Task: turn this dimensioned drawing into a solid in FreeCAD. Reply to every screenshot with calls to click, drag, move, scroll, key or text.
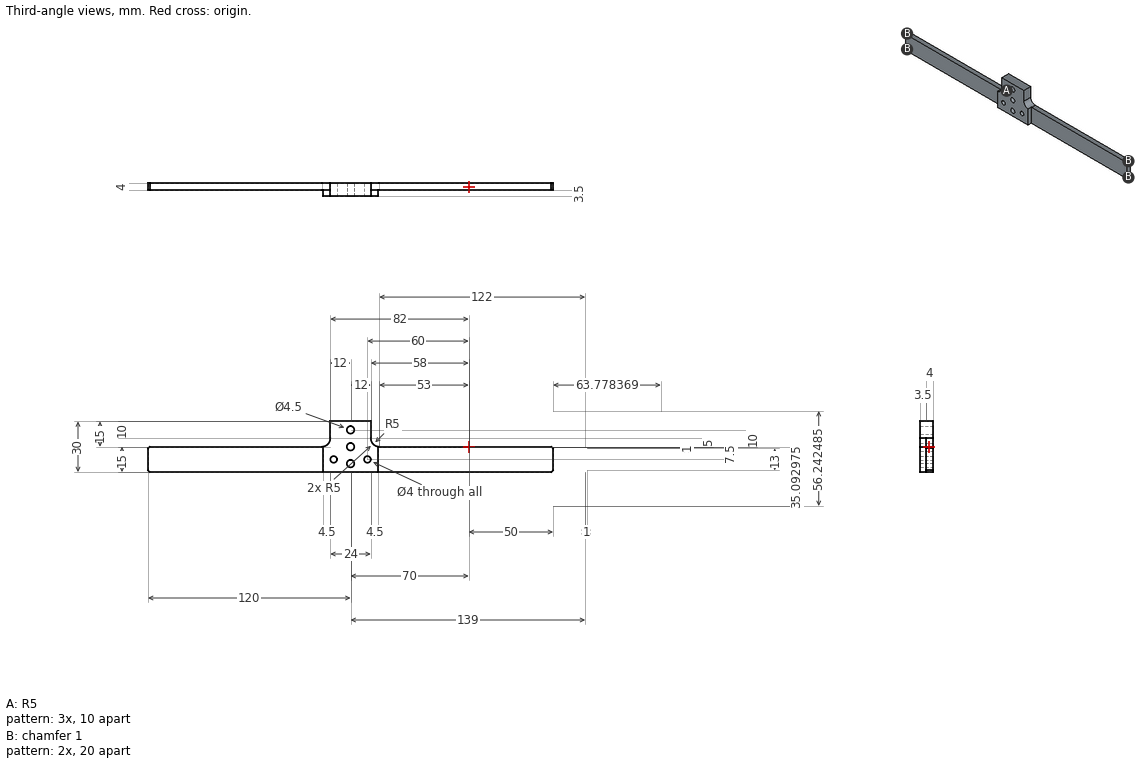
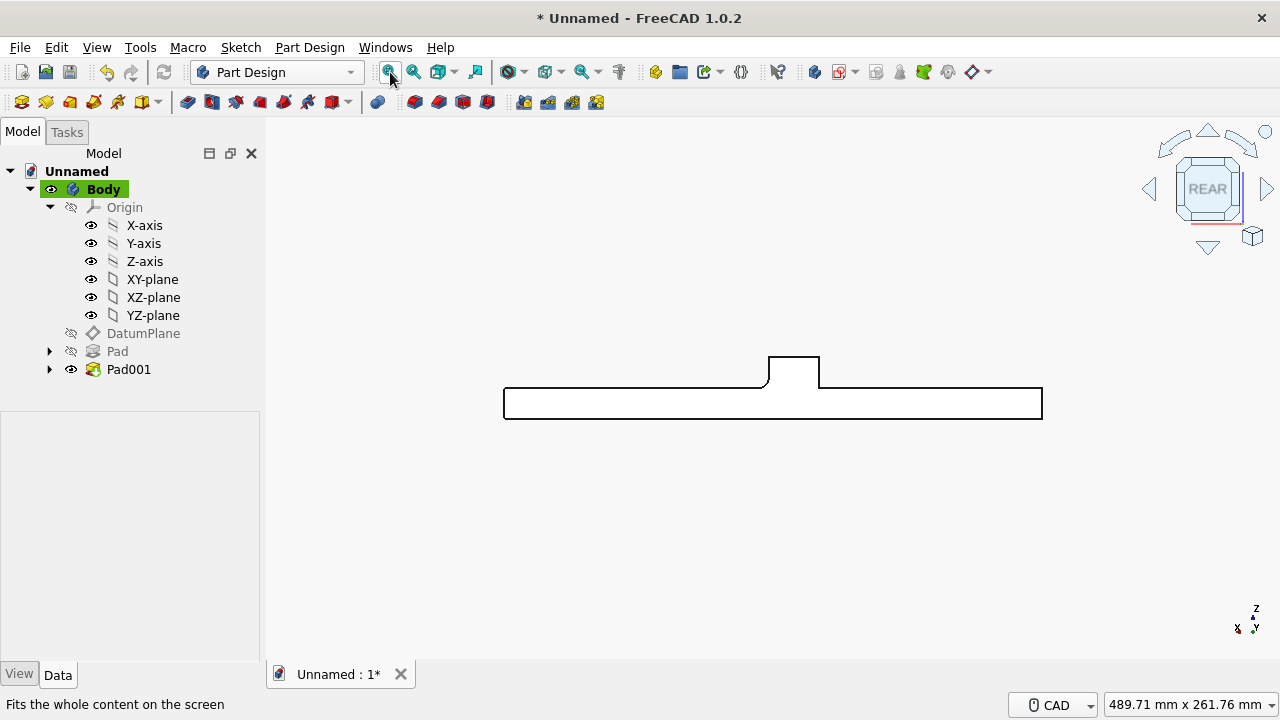
scroll(819, 387, up, 8)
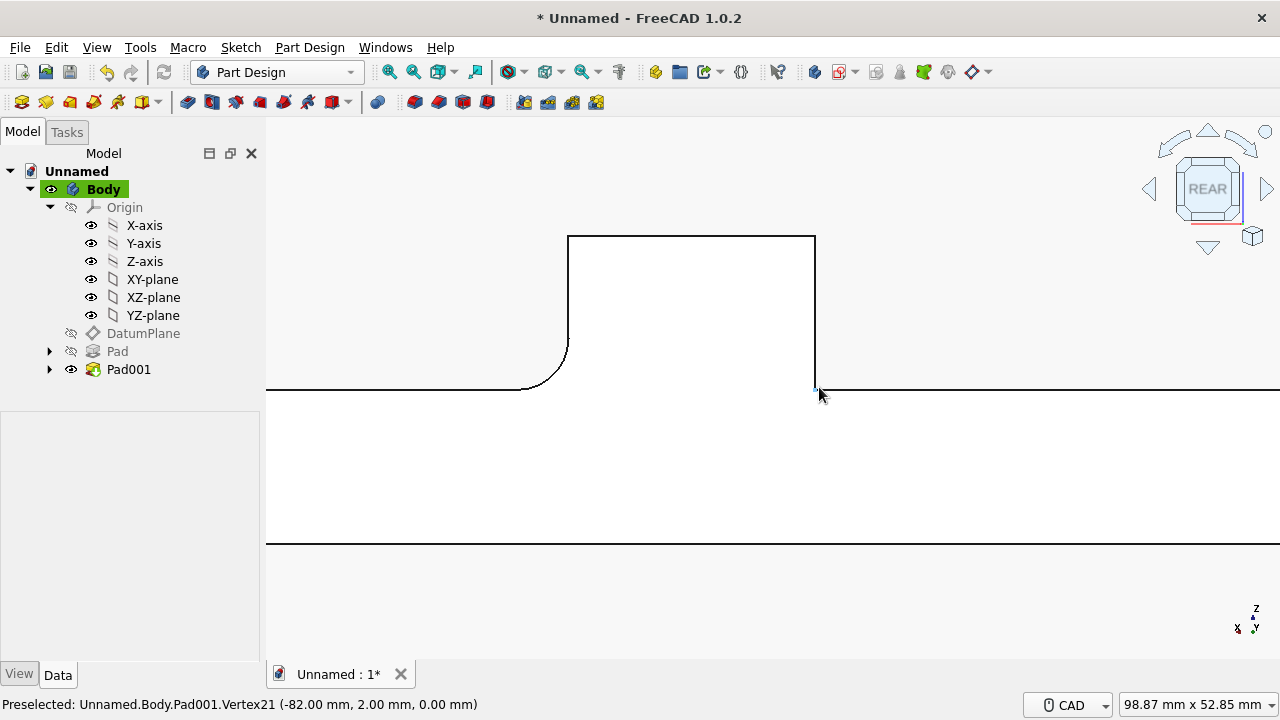
click(390, 72)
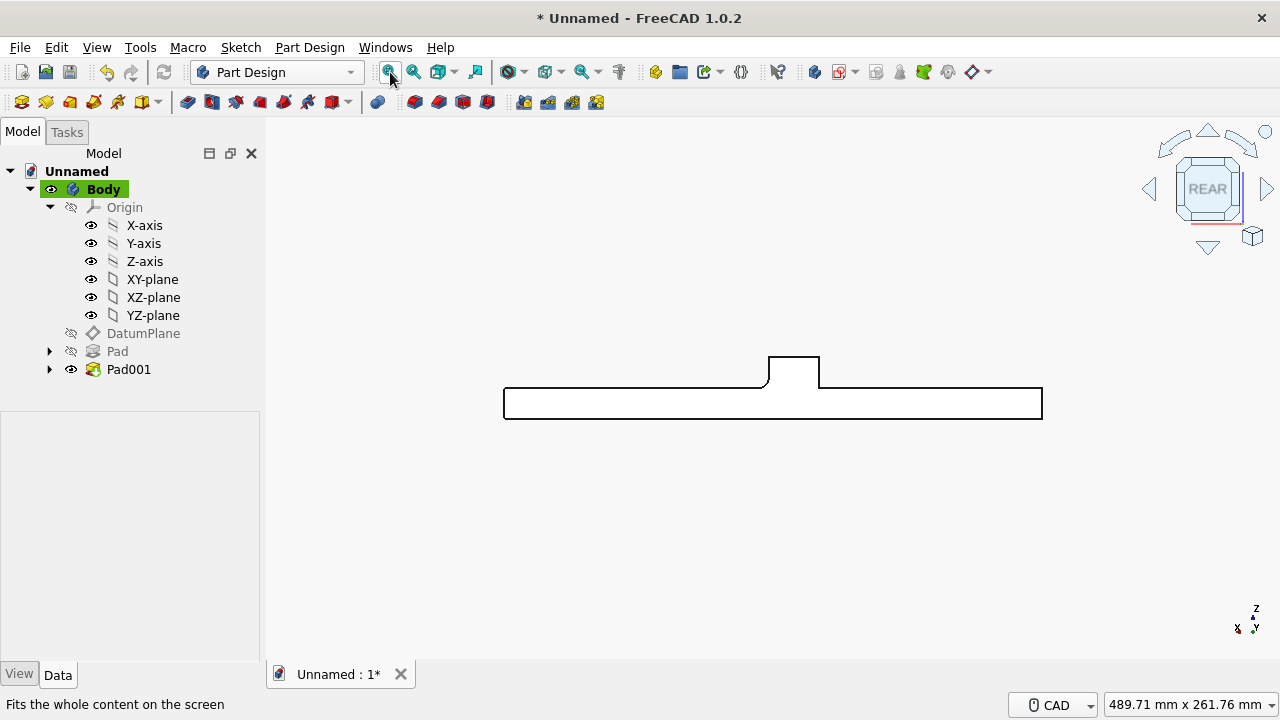
key(6)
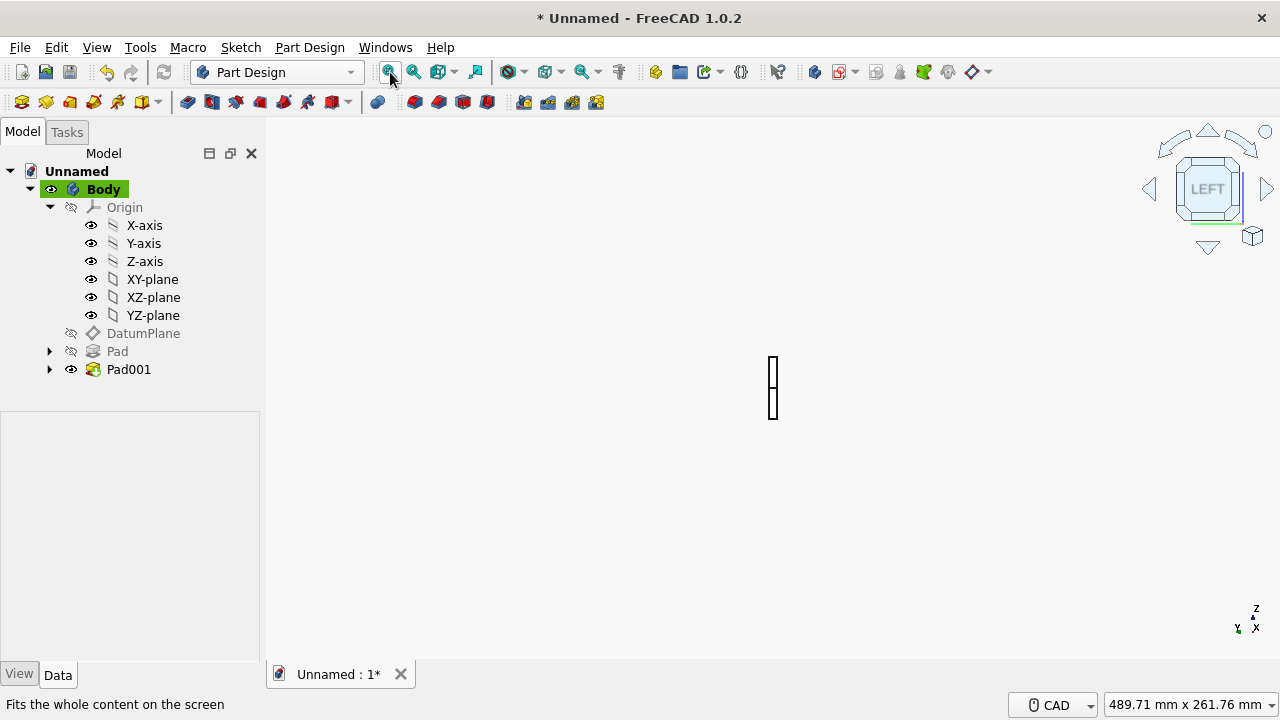
click(390, 72)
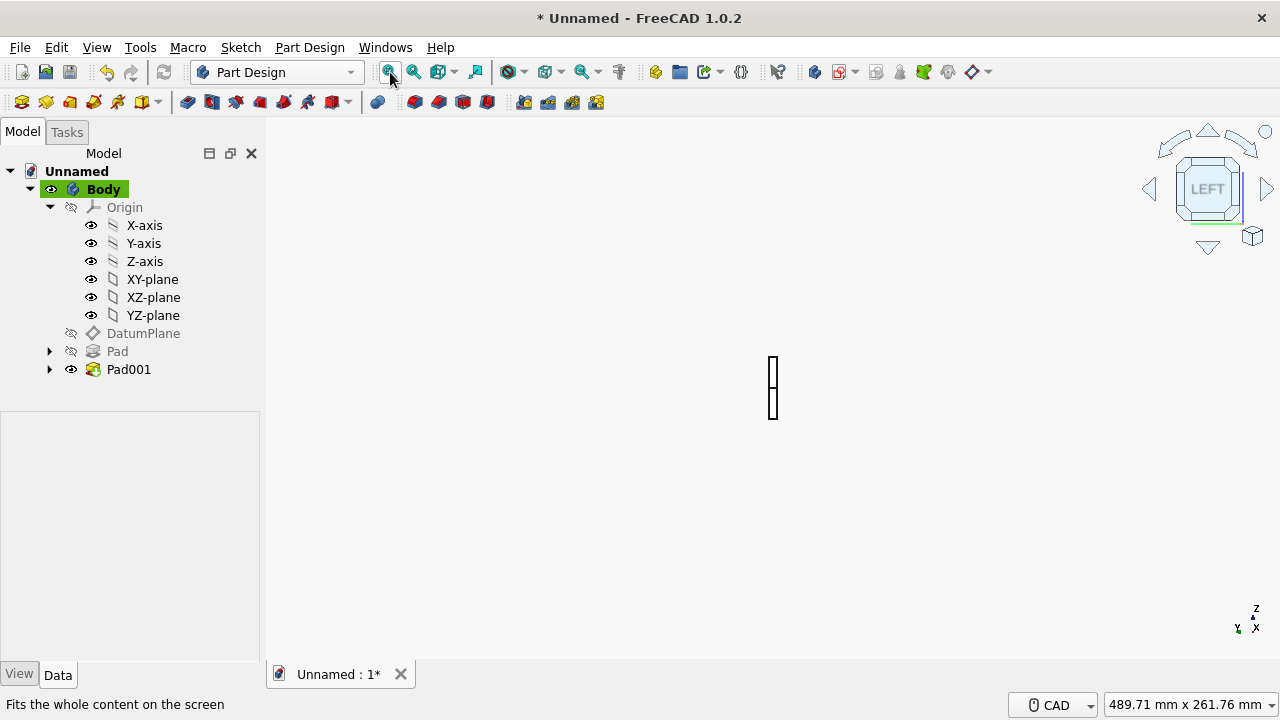
scroll(773, 387, up, 8)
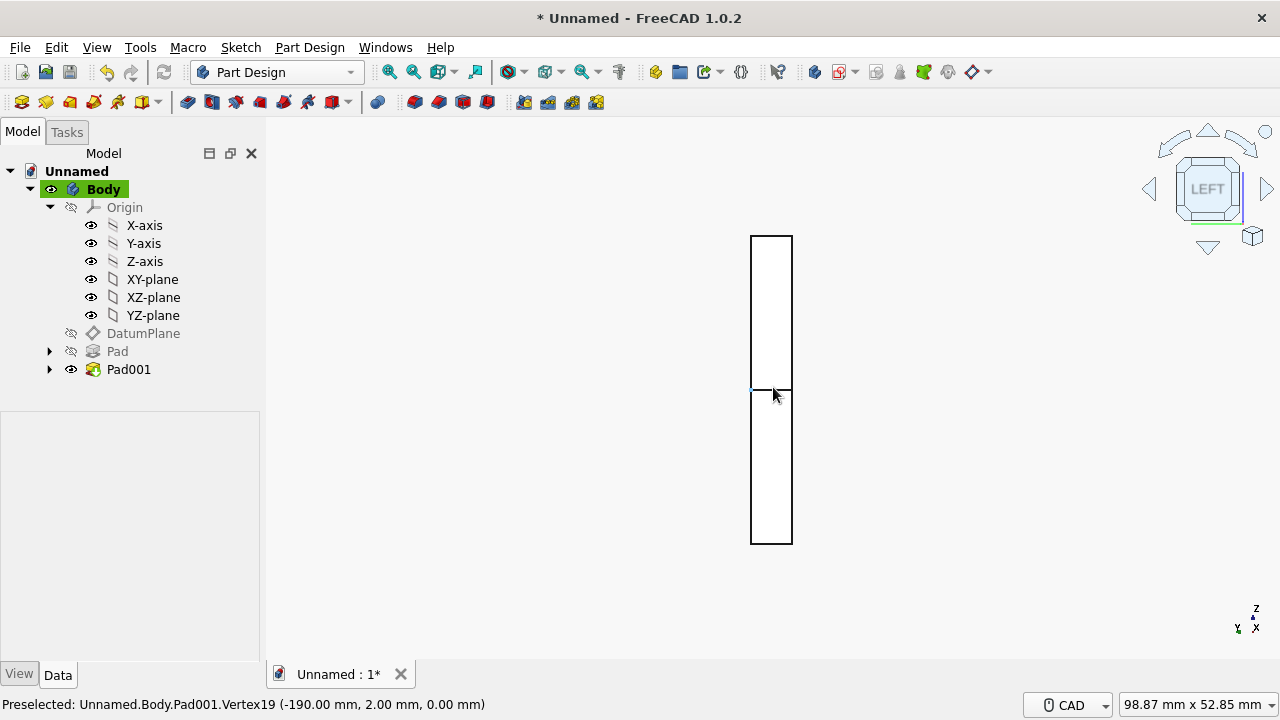
click(390, 72)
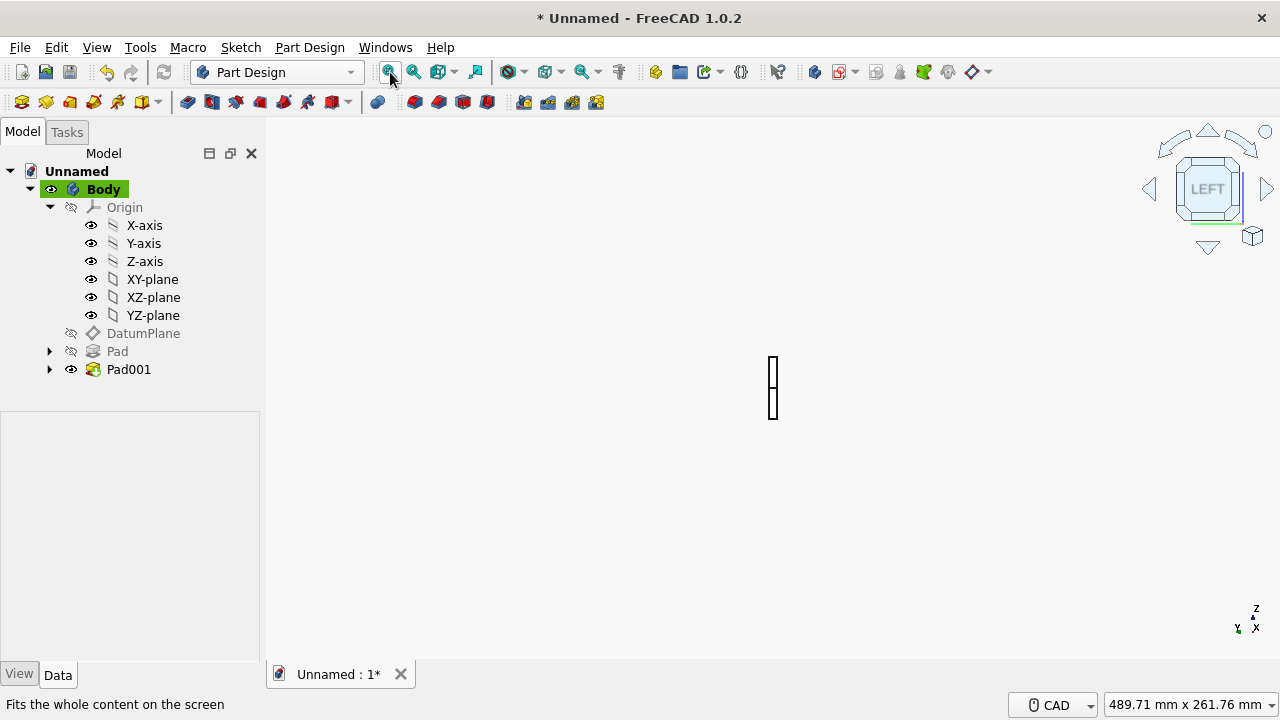
key(v)
key(3)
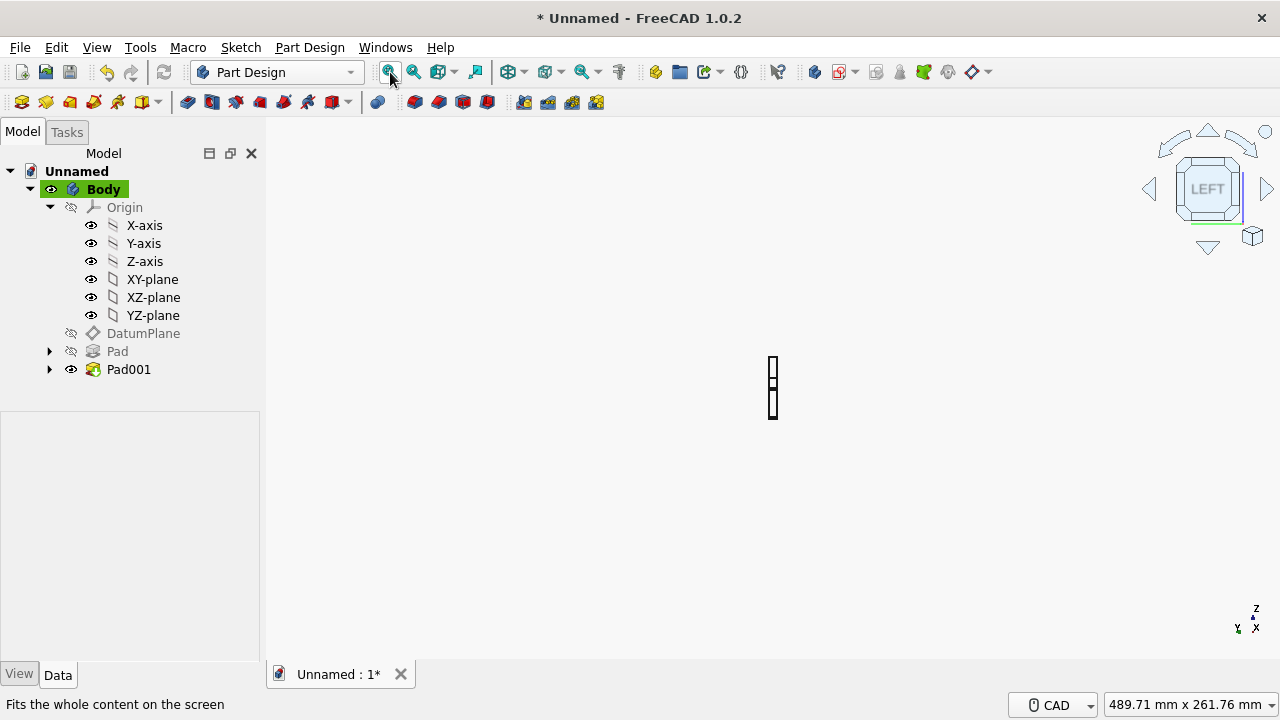
key(0)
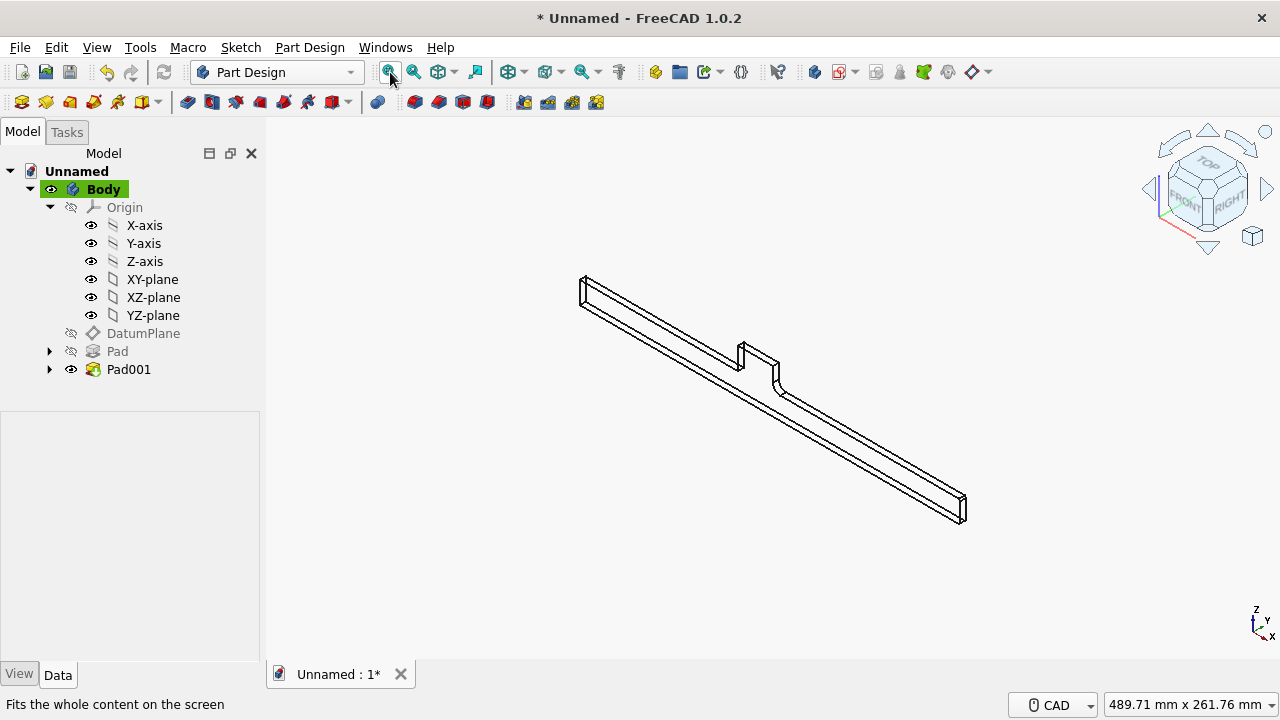
scroll(741, 368, up, 8)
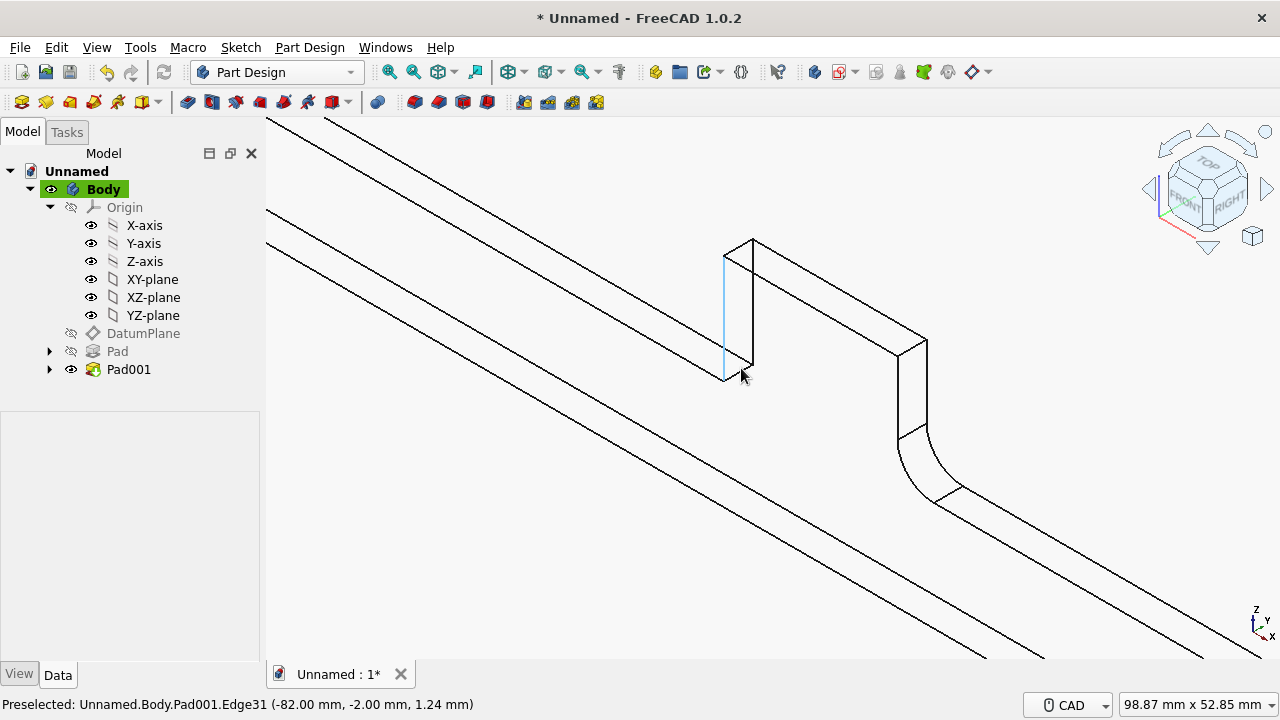
click(738, 372)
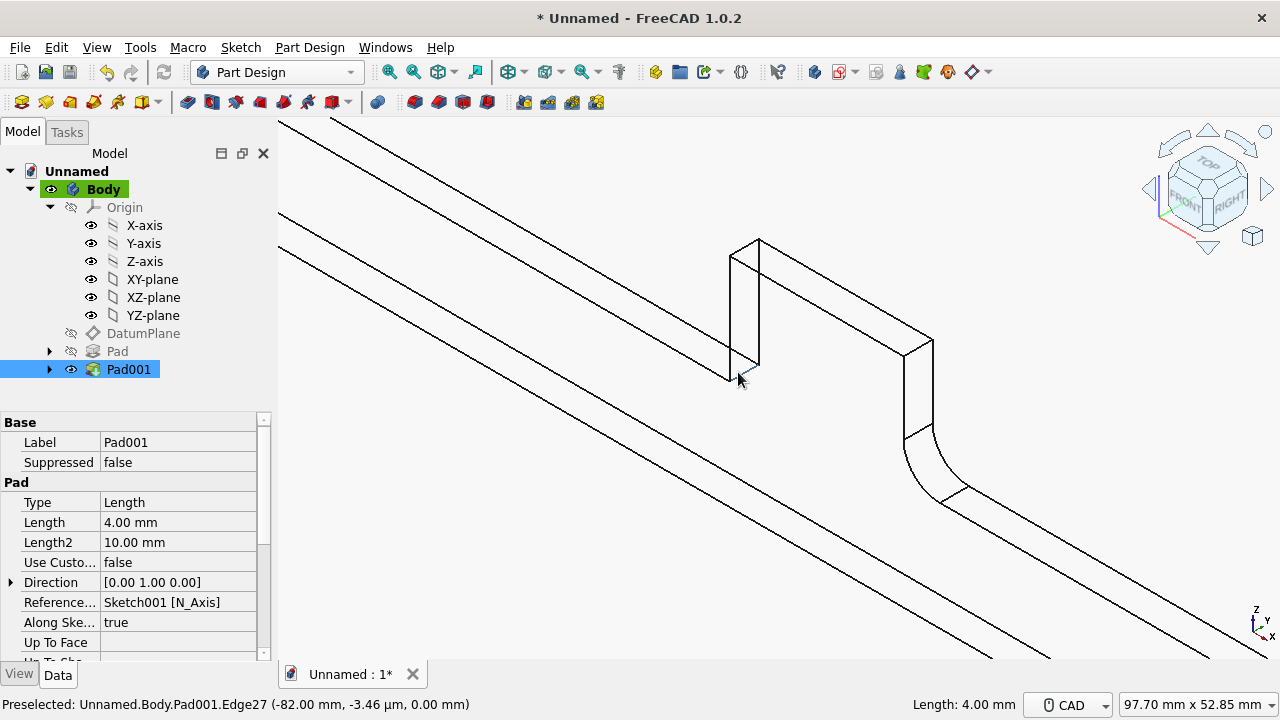
key(v)
key(1)